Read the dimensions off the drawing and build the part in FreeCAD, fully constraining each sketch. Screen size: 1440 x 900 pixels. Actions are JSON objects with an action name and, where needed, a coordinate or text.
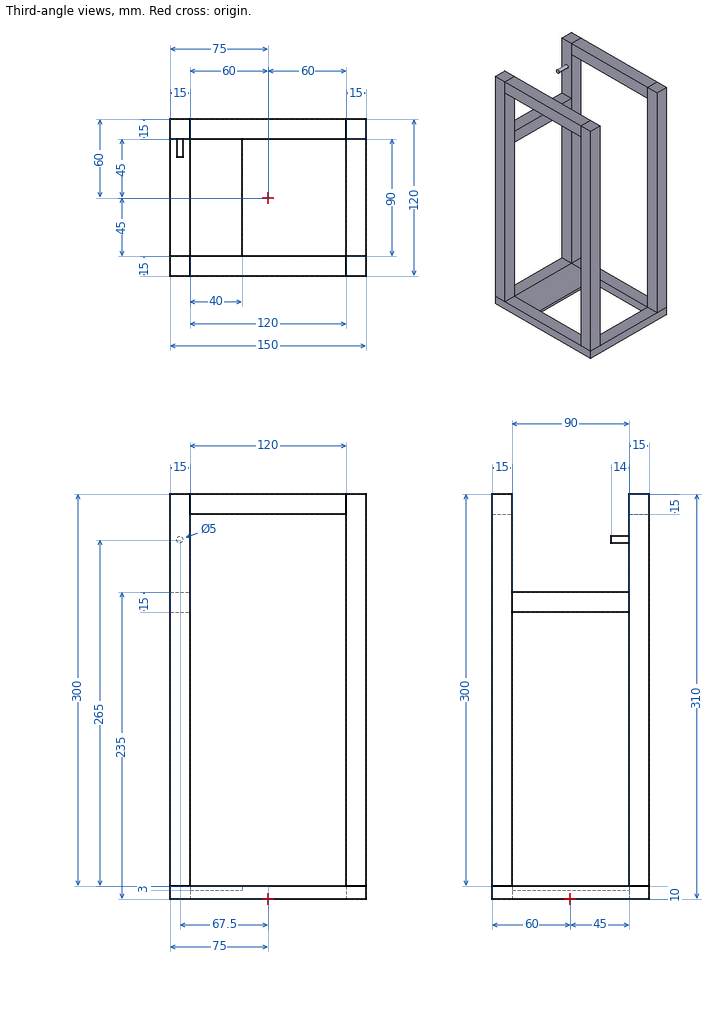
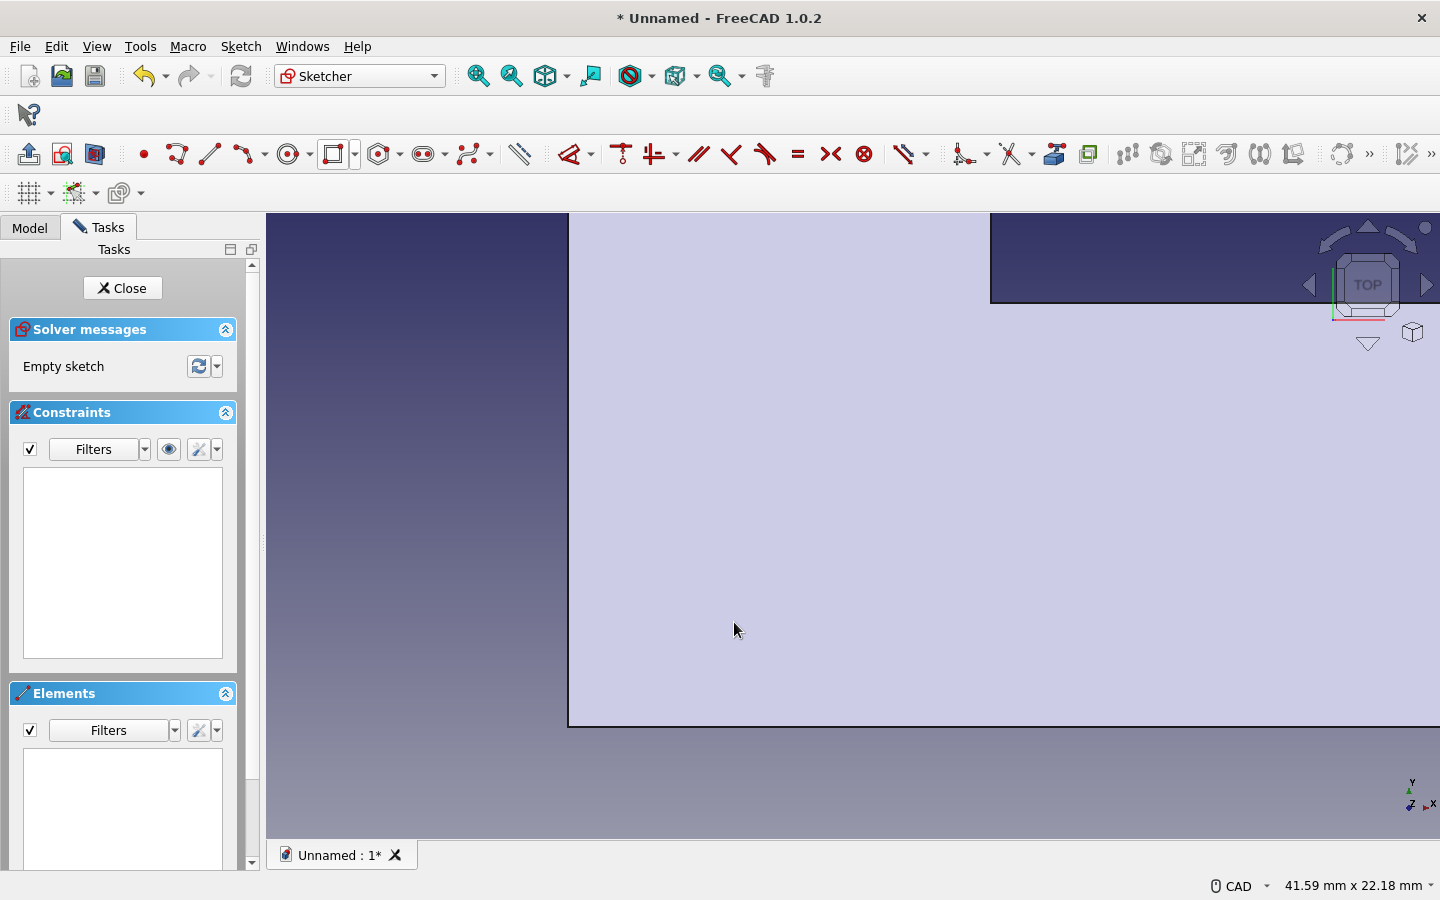
{"action": "left_click", "coordinate": [332, 154]}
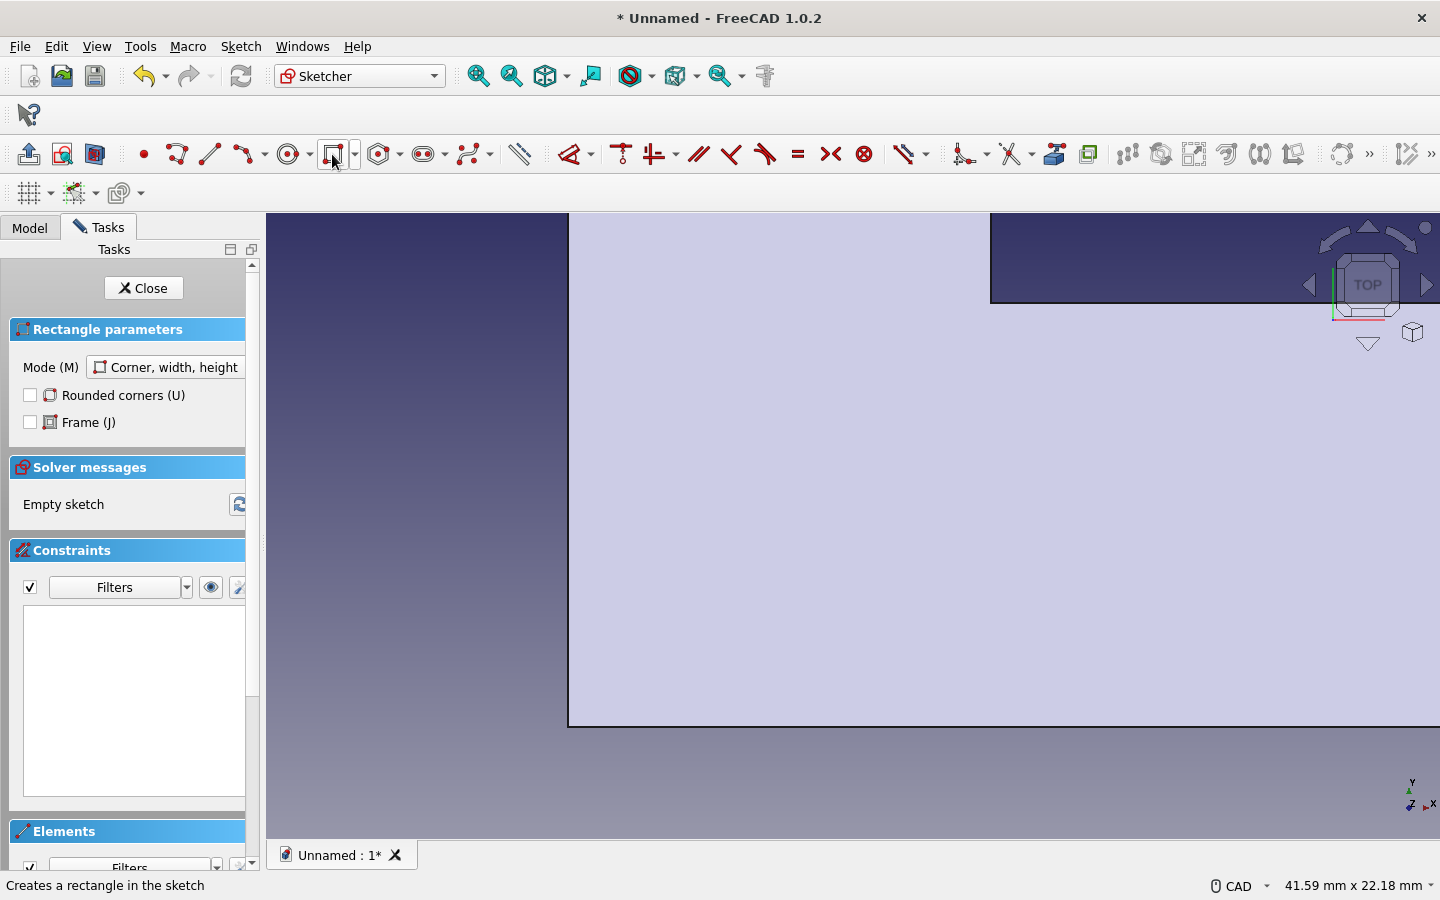
{"action": "left_click", "coordinate": [568, 303]}
{"action": "left_click", "coordinate": [991, 727]}
{"action": "key", "text": "Escape"}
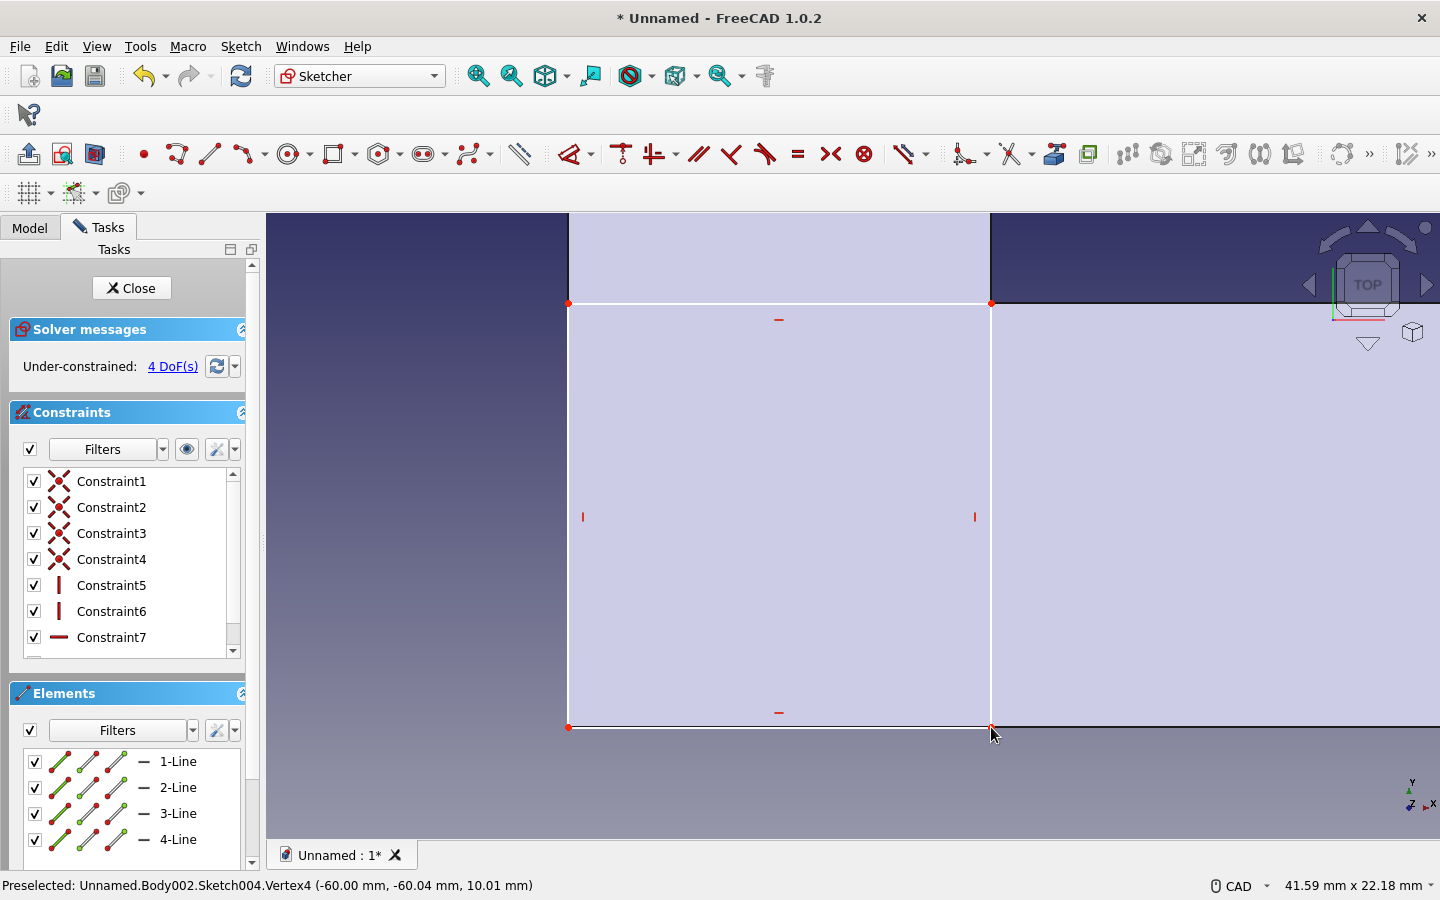
{"action": "left_click", "coordinate": [568, 154]}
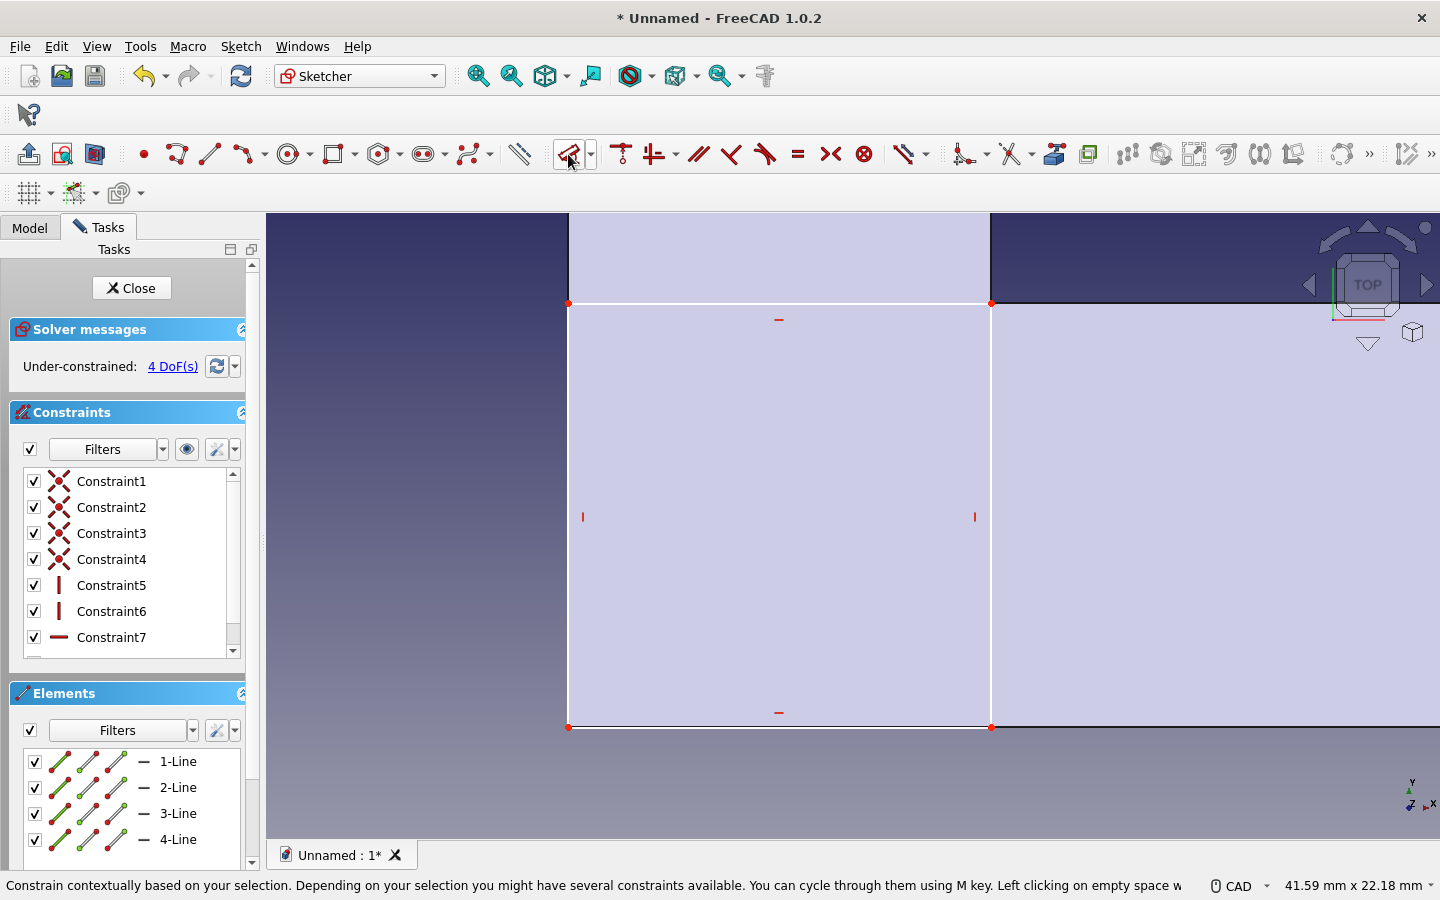
{"action": "left_click", "coordinate": [568, 431]}
{"action": "left_click", "coordinate": [534, 516]}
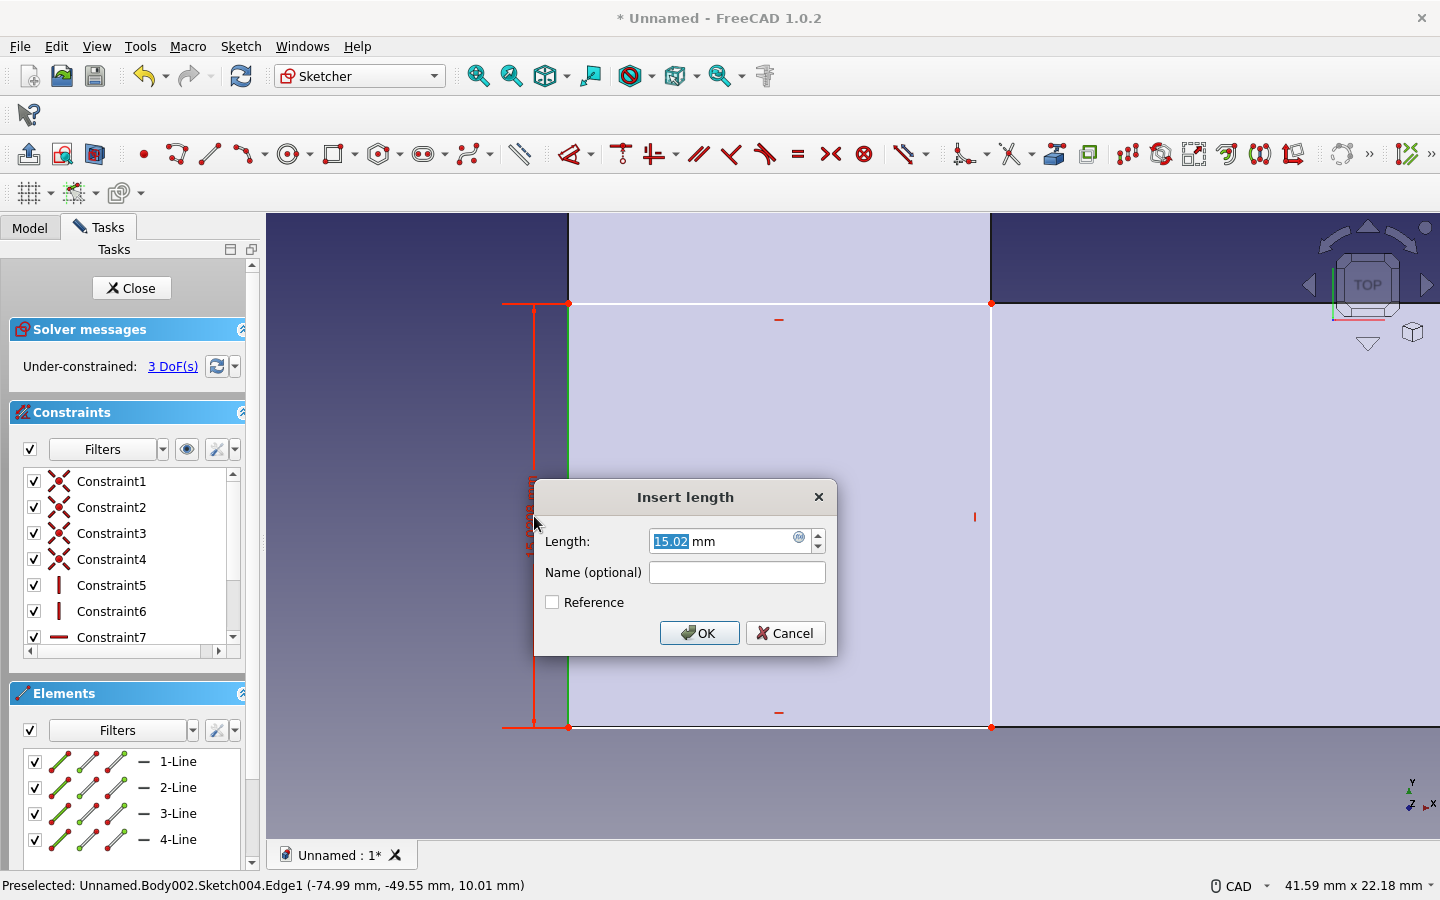
{"action": "type", "text": "15"}
{"action": "key", "text": "Return"}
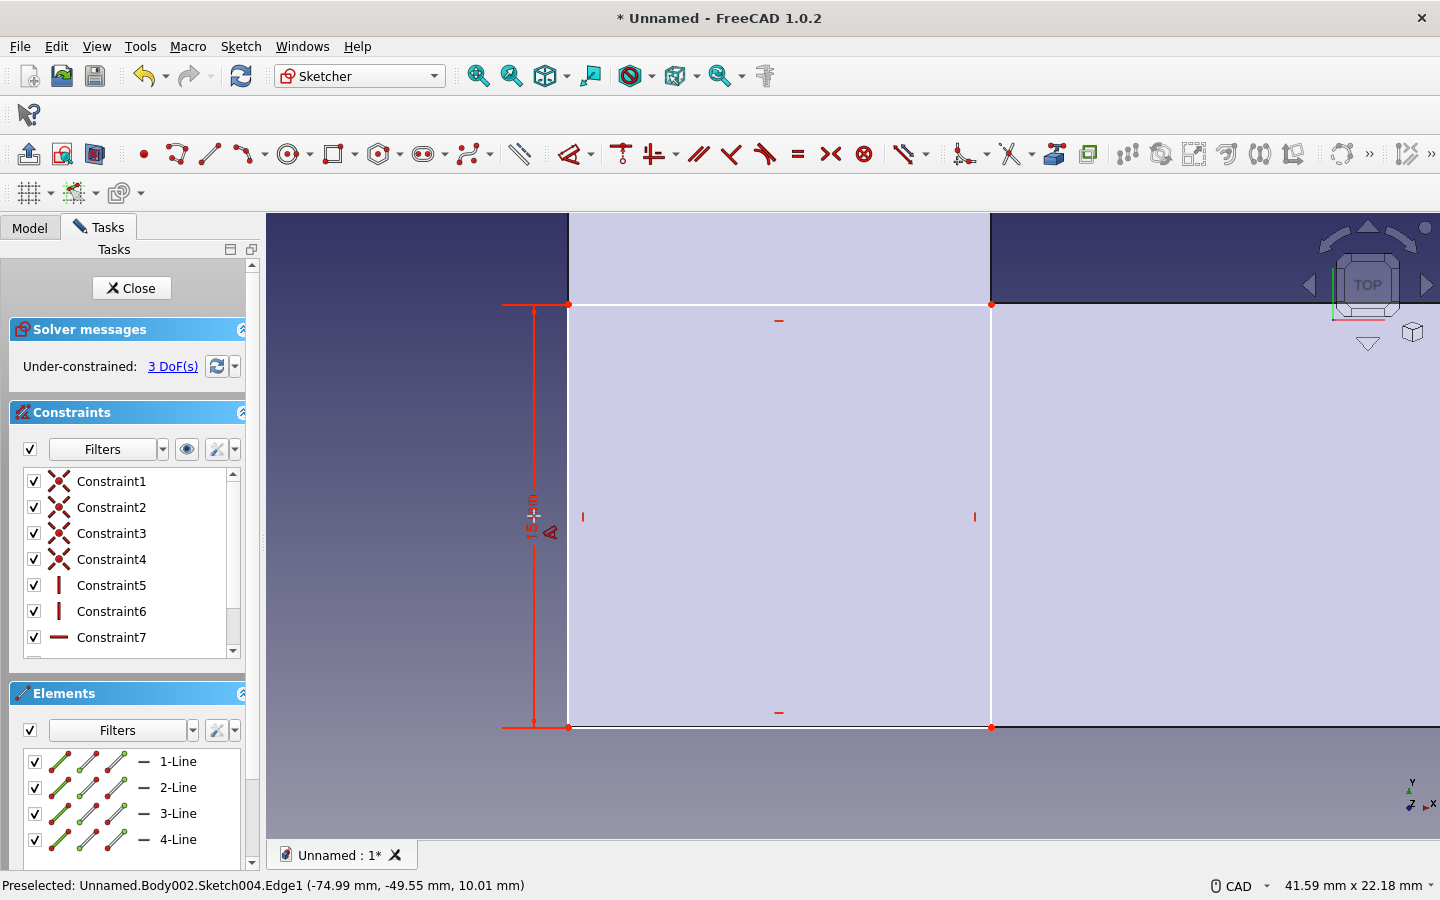
{"action": "left_click", "coordinate": [695, 728]}
{"action": "left_click", "coordinate": [779, 762]}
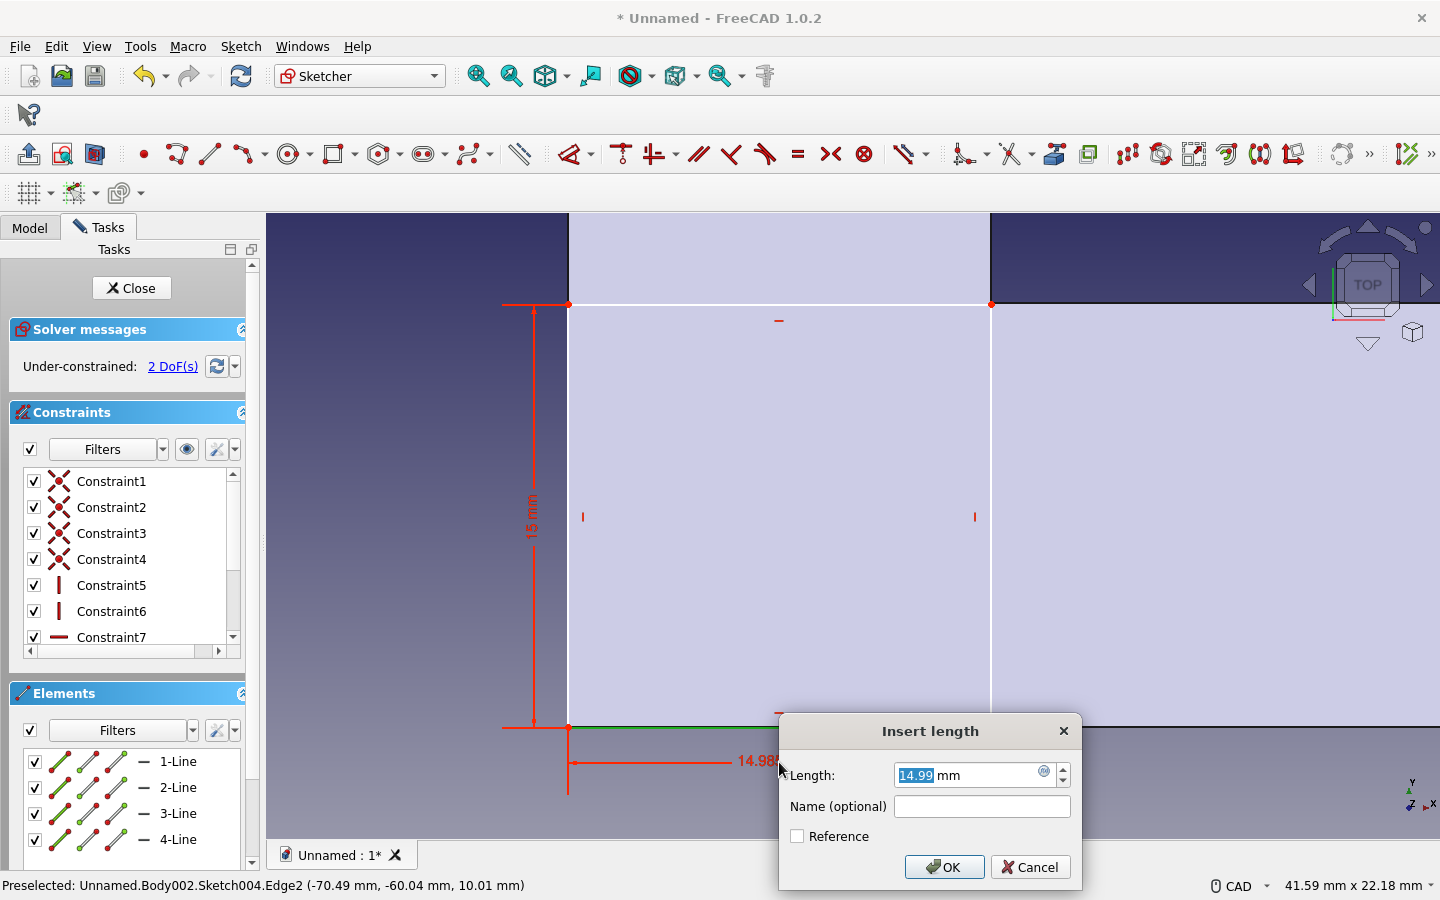
{"action": "type", "text": "15"}
{"action": "key", "text": "Return"}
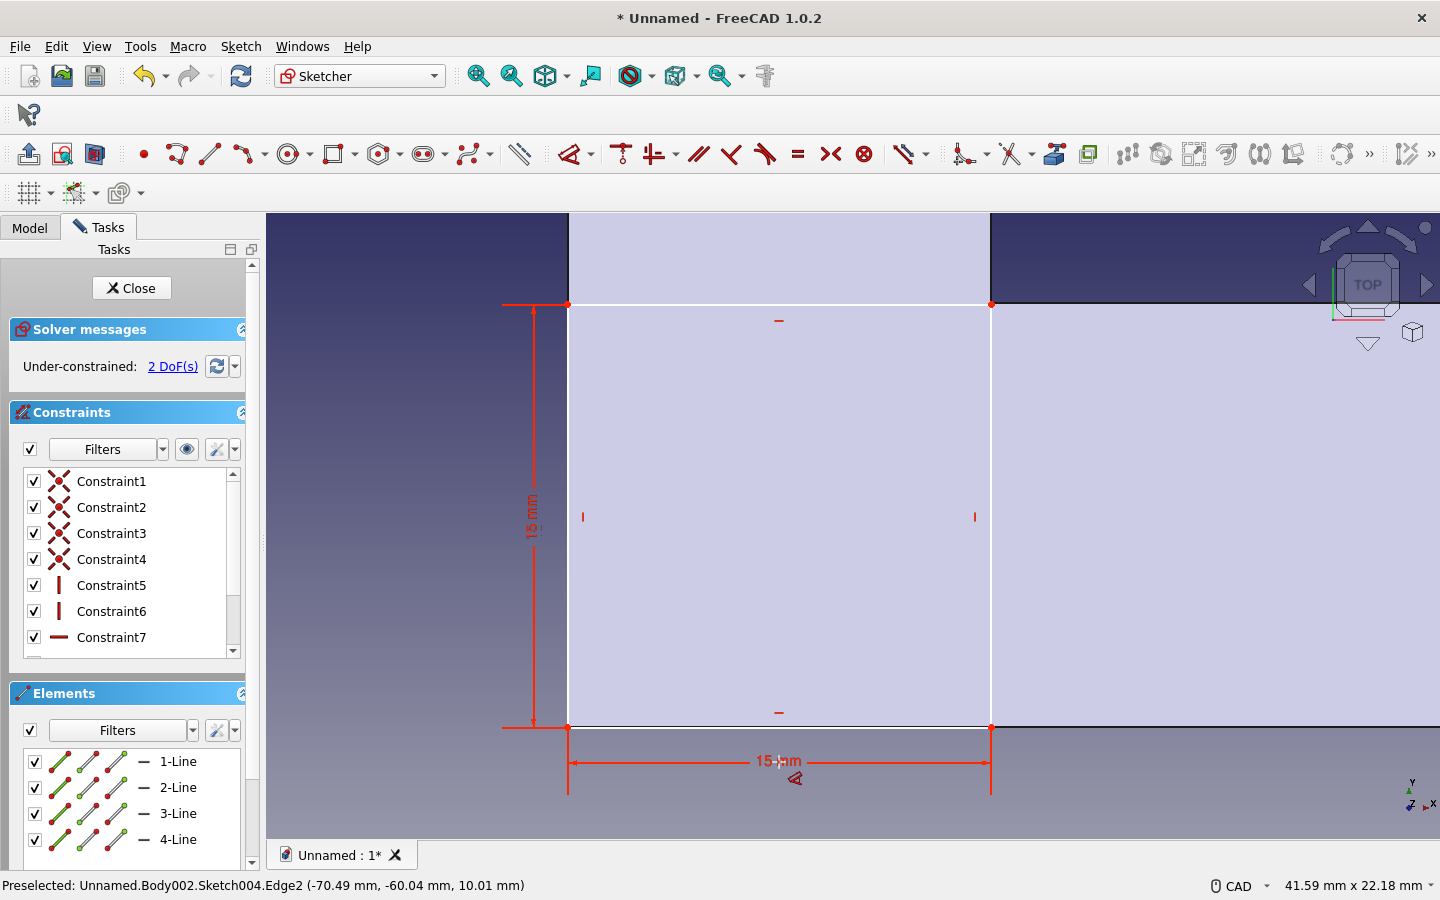
{"action": "left_click", "coordinate": [568, 305]}
{"action": "left_click", "coordinate": [921, 339]}